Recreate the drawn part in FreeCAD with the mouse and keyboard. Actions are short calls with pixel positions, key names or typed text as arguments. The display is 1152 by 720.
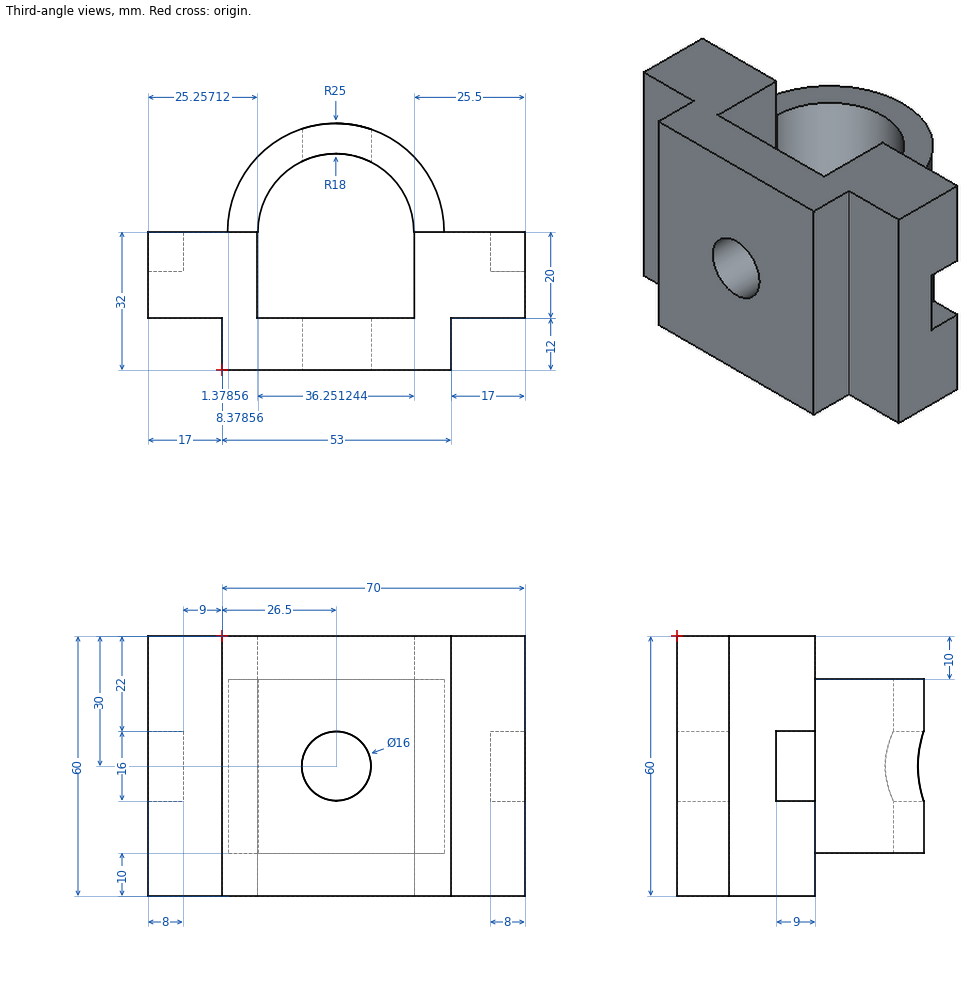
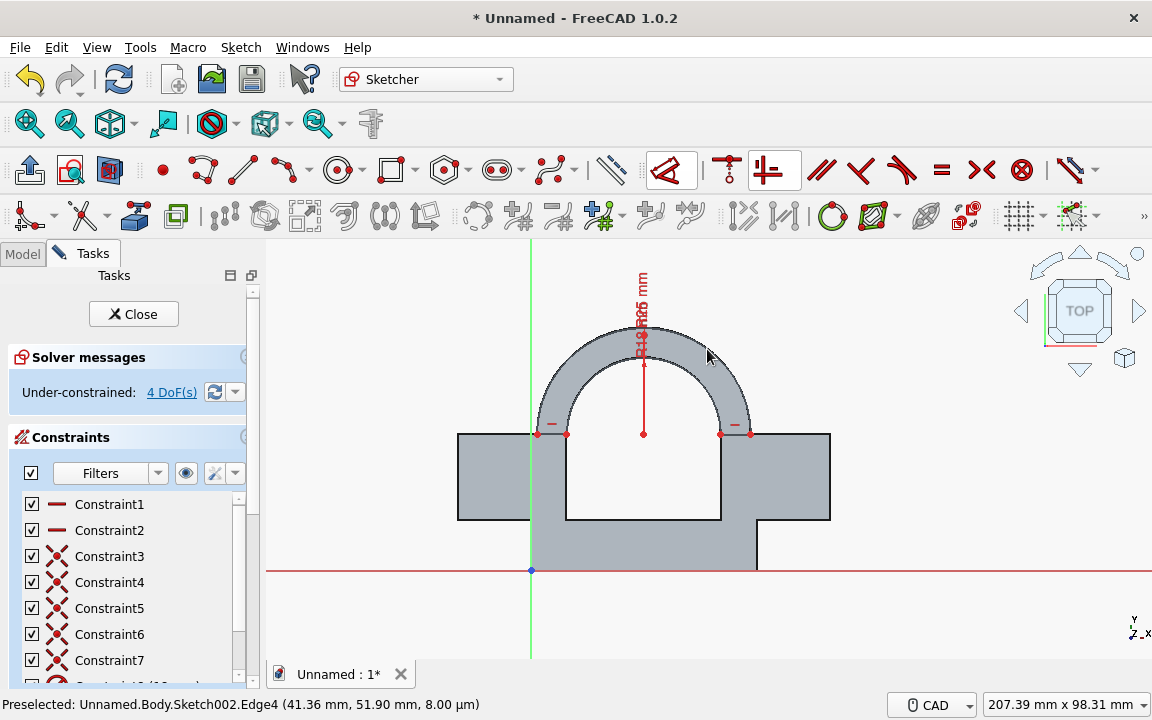
click(537, 434)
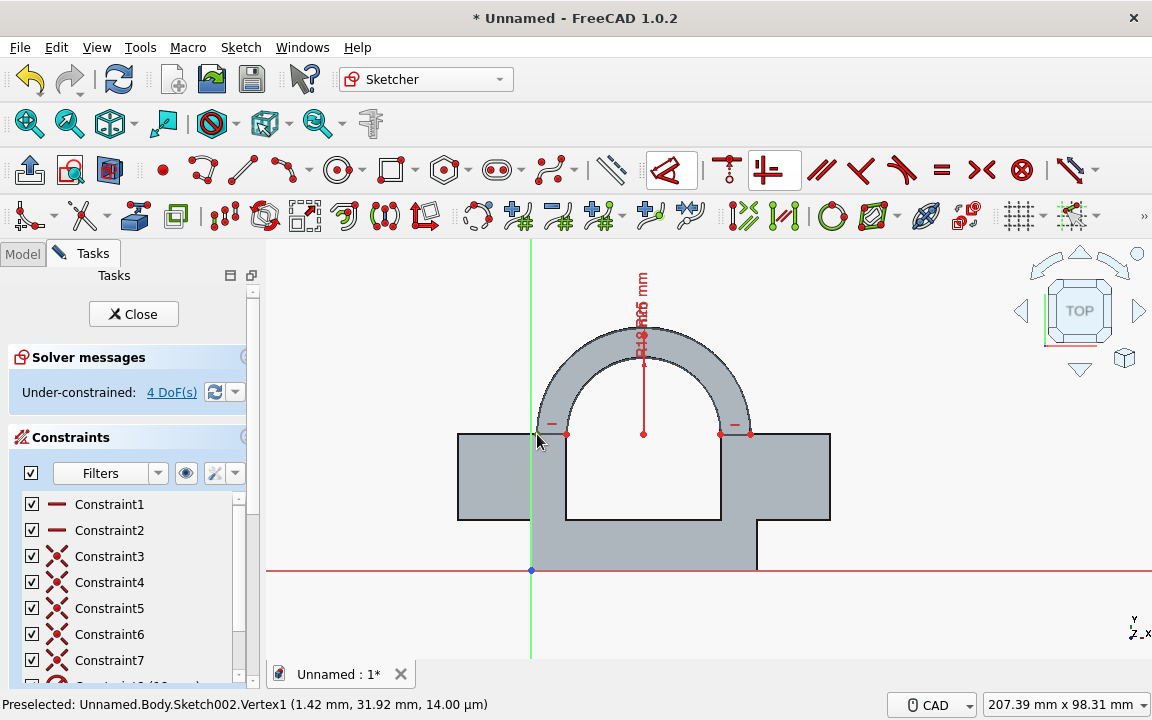
click(692, 170)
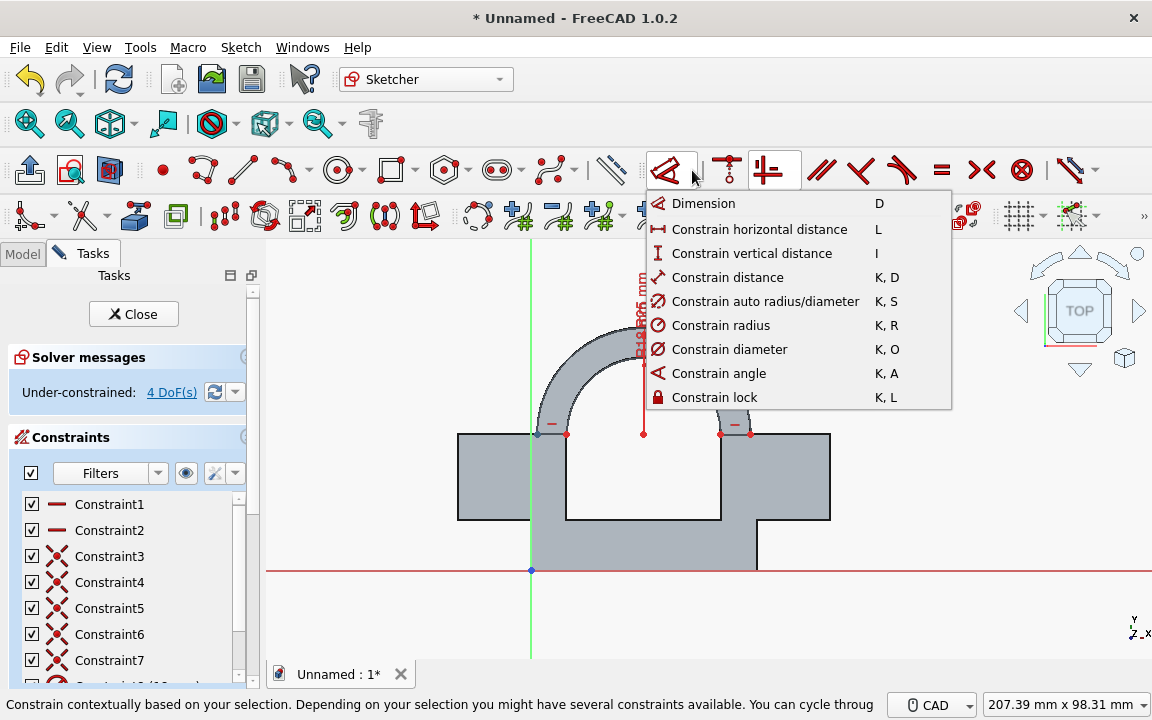
click(799, 253)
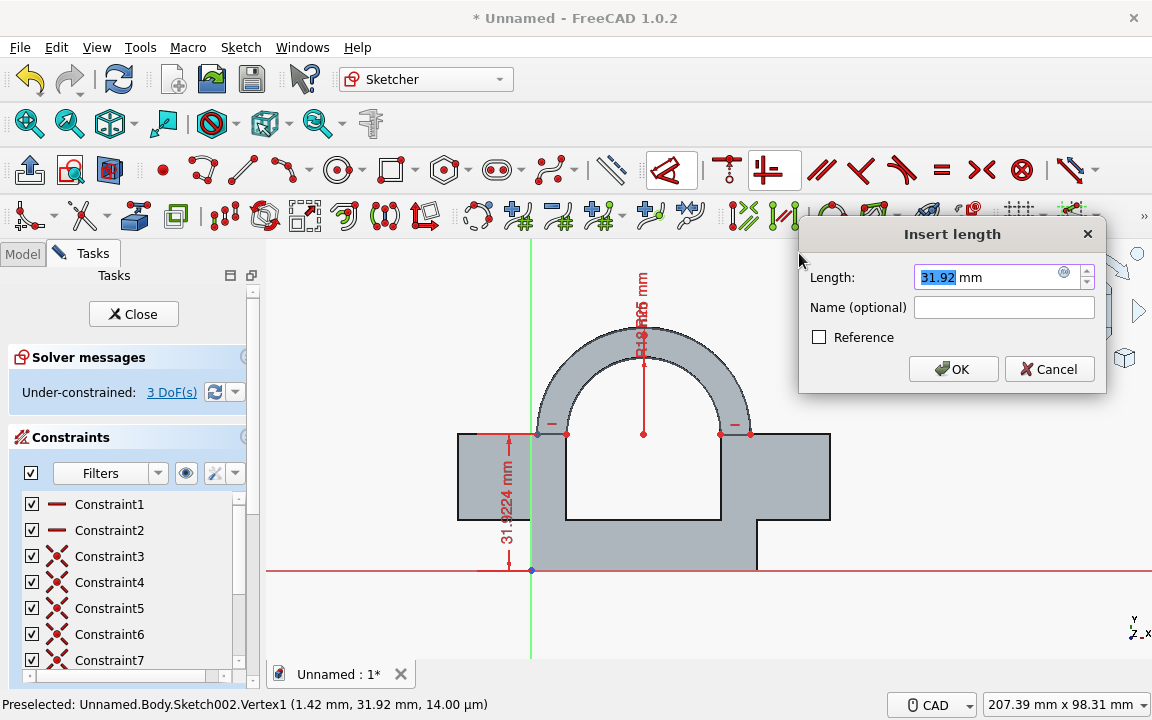
text(32)
key(Return)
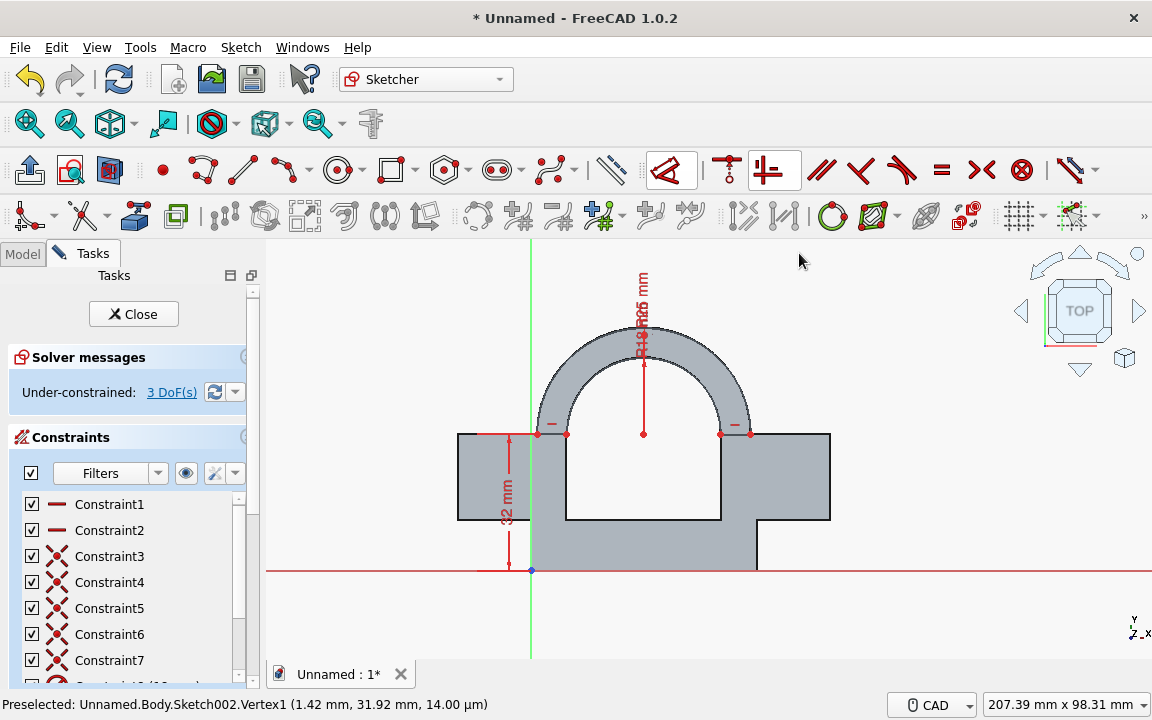
click(721, 435)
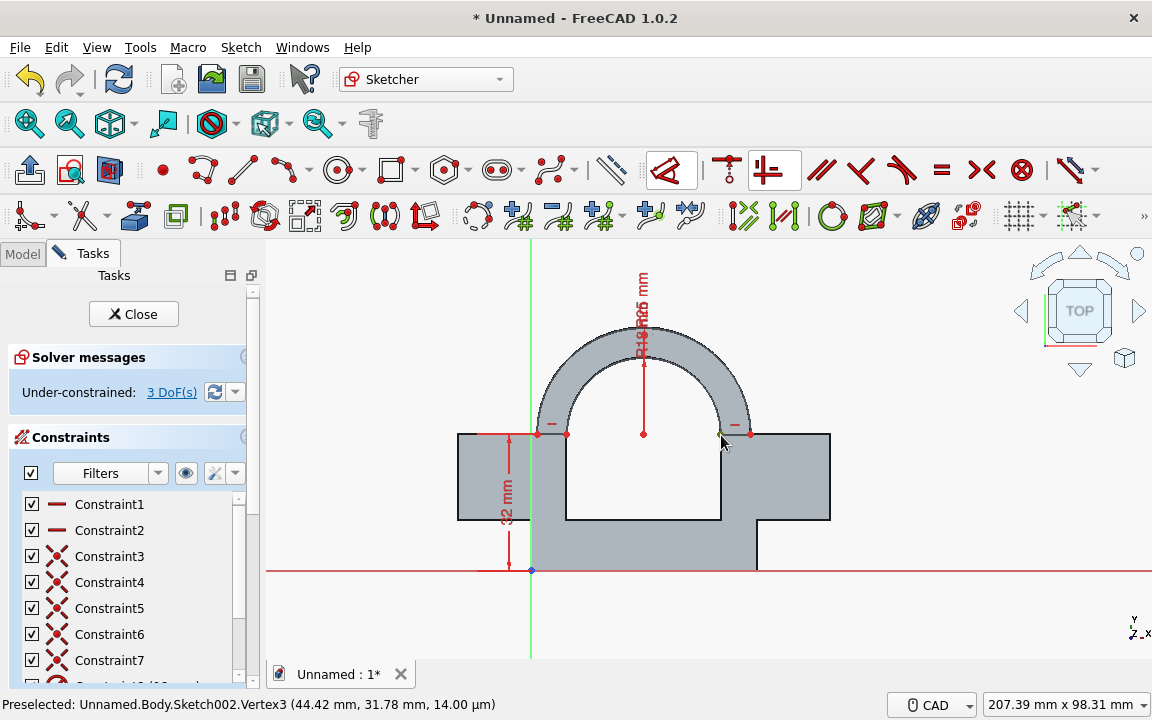
key(i)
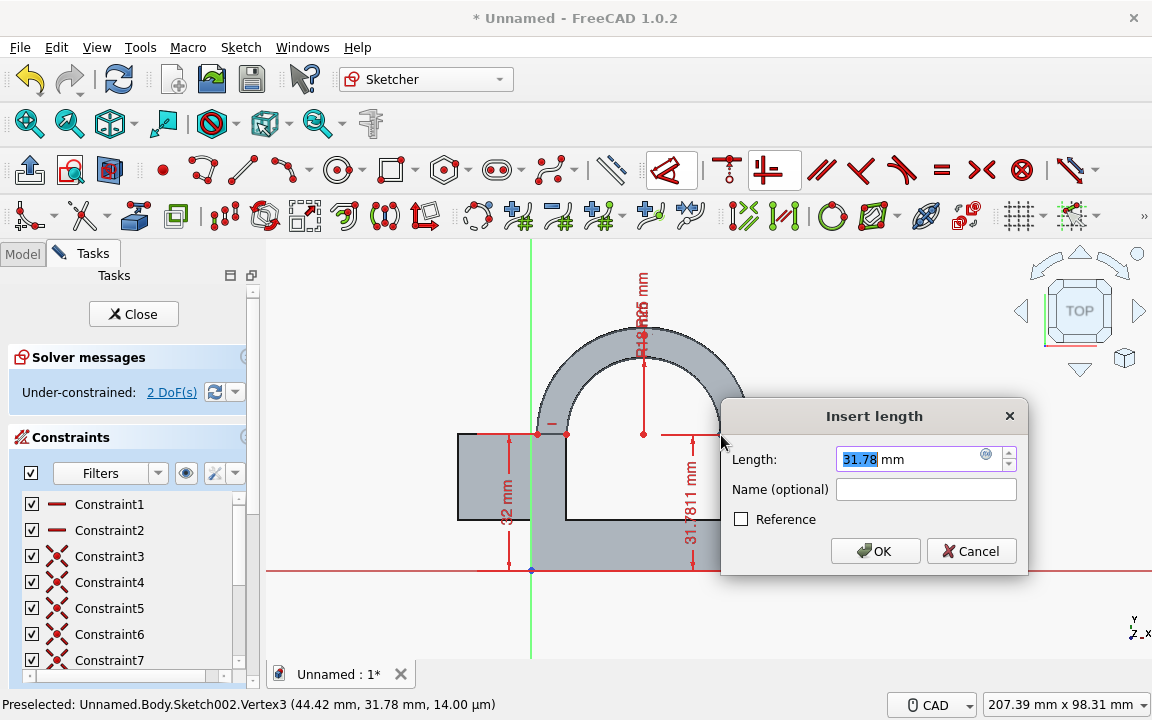
text(32)
key(Return)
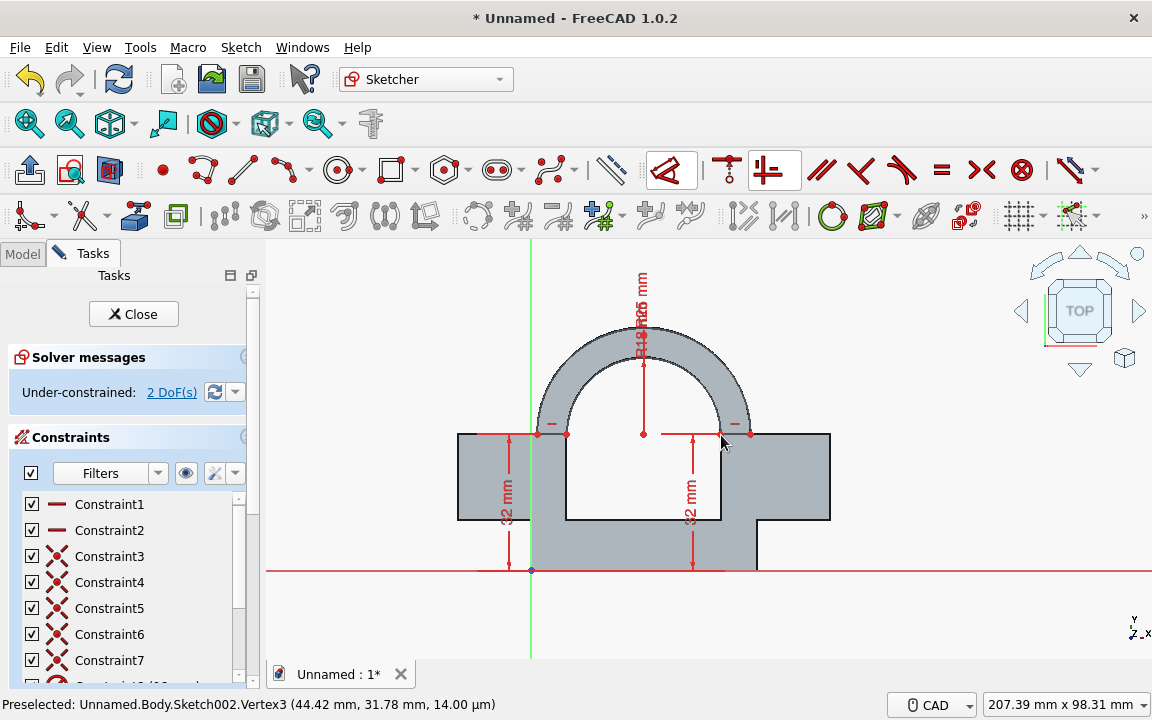
click(644, 435)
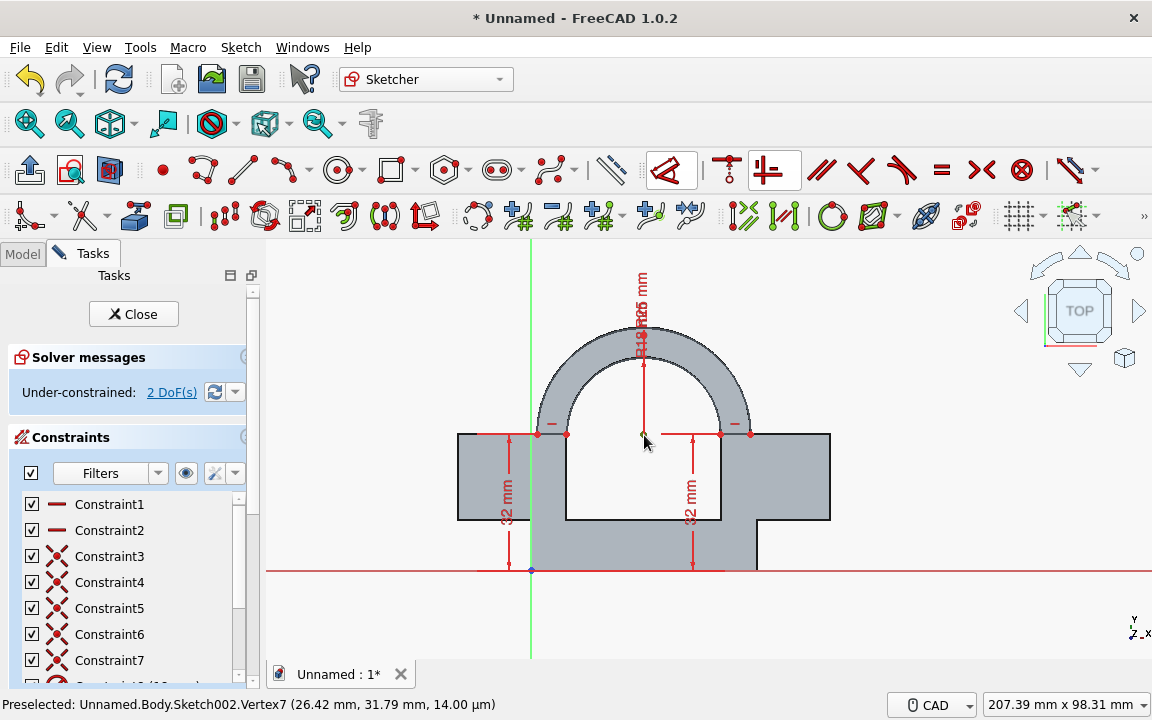
click(692, 170)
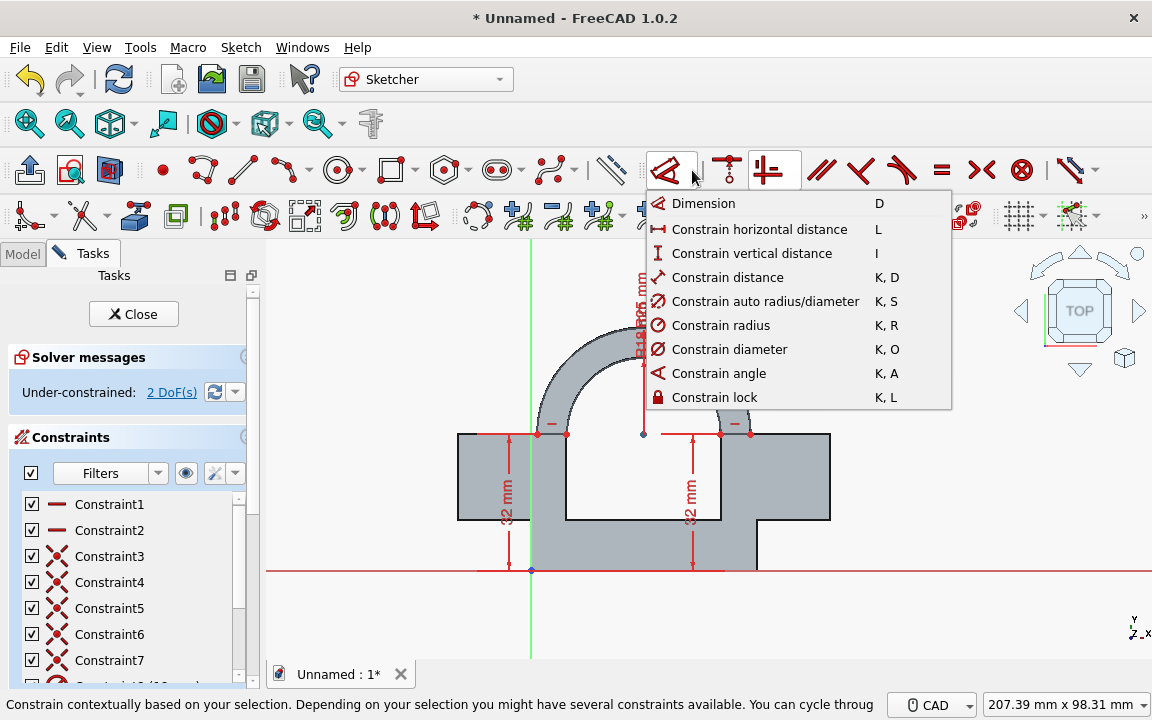
click(799, 253)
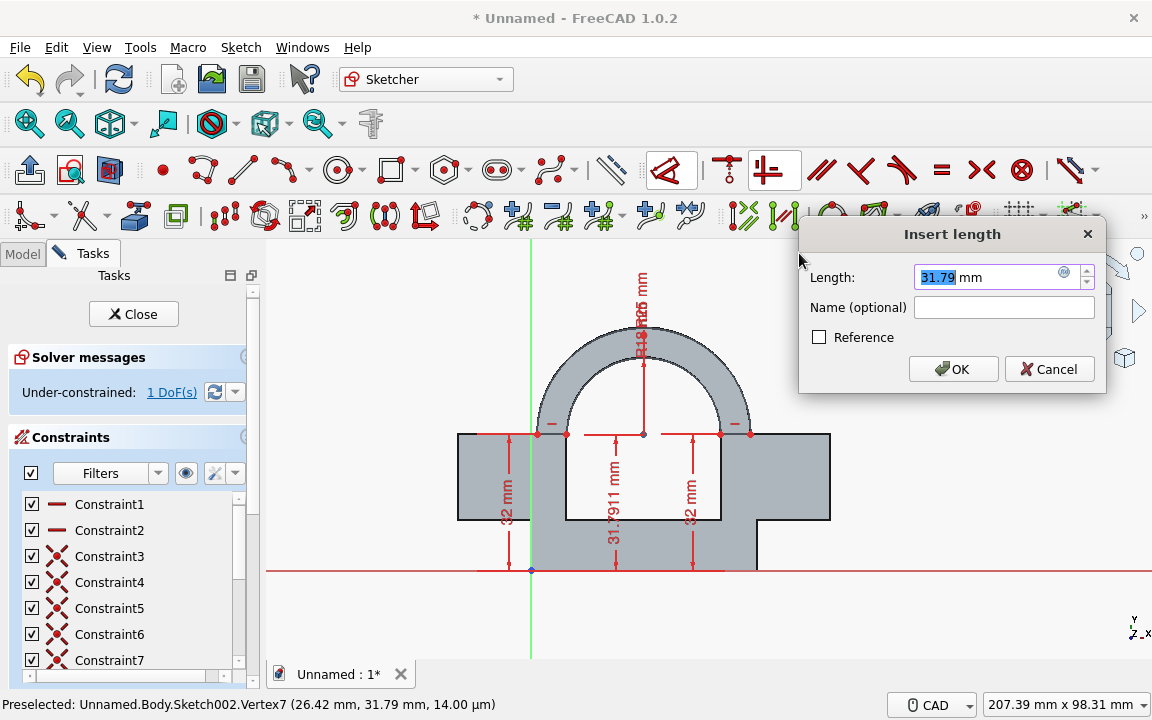
text(32)
key(Return)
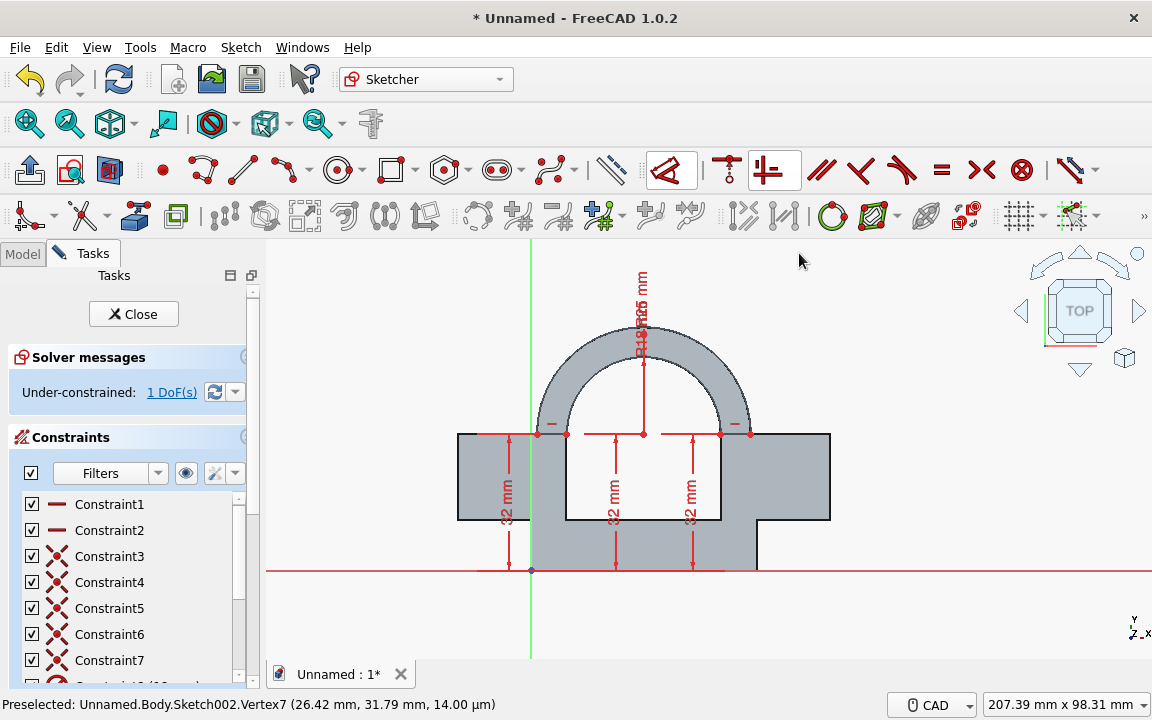
scroll(537, 434, up, 10)